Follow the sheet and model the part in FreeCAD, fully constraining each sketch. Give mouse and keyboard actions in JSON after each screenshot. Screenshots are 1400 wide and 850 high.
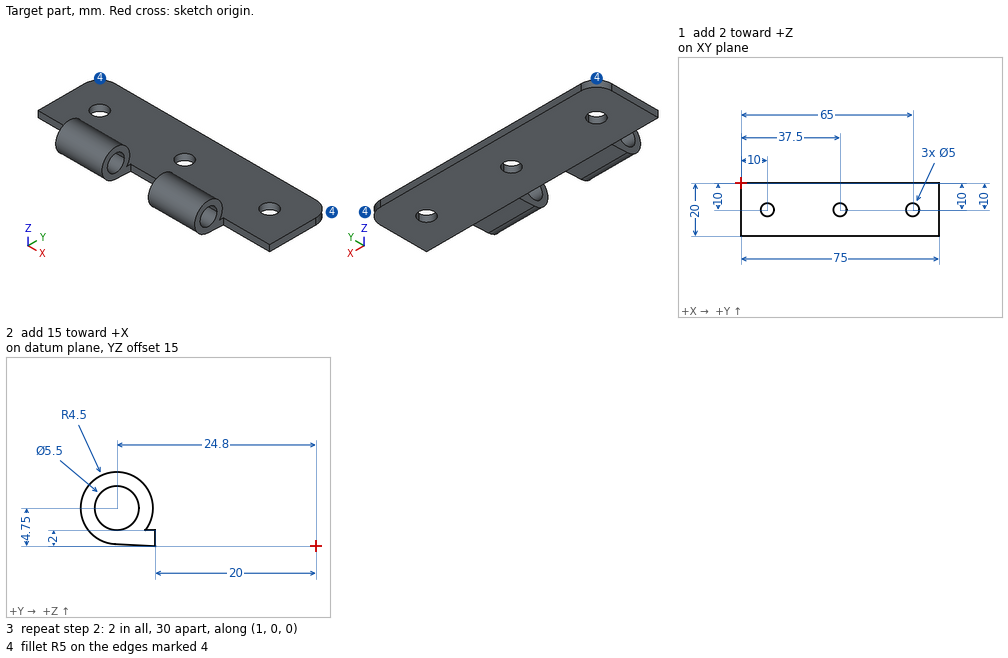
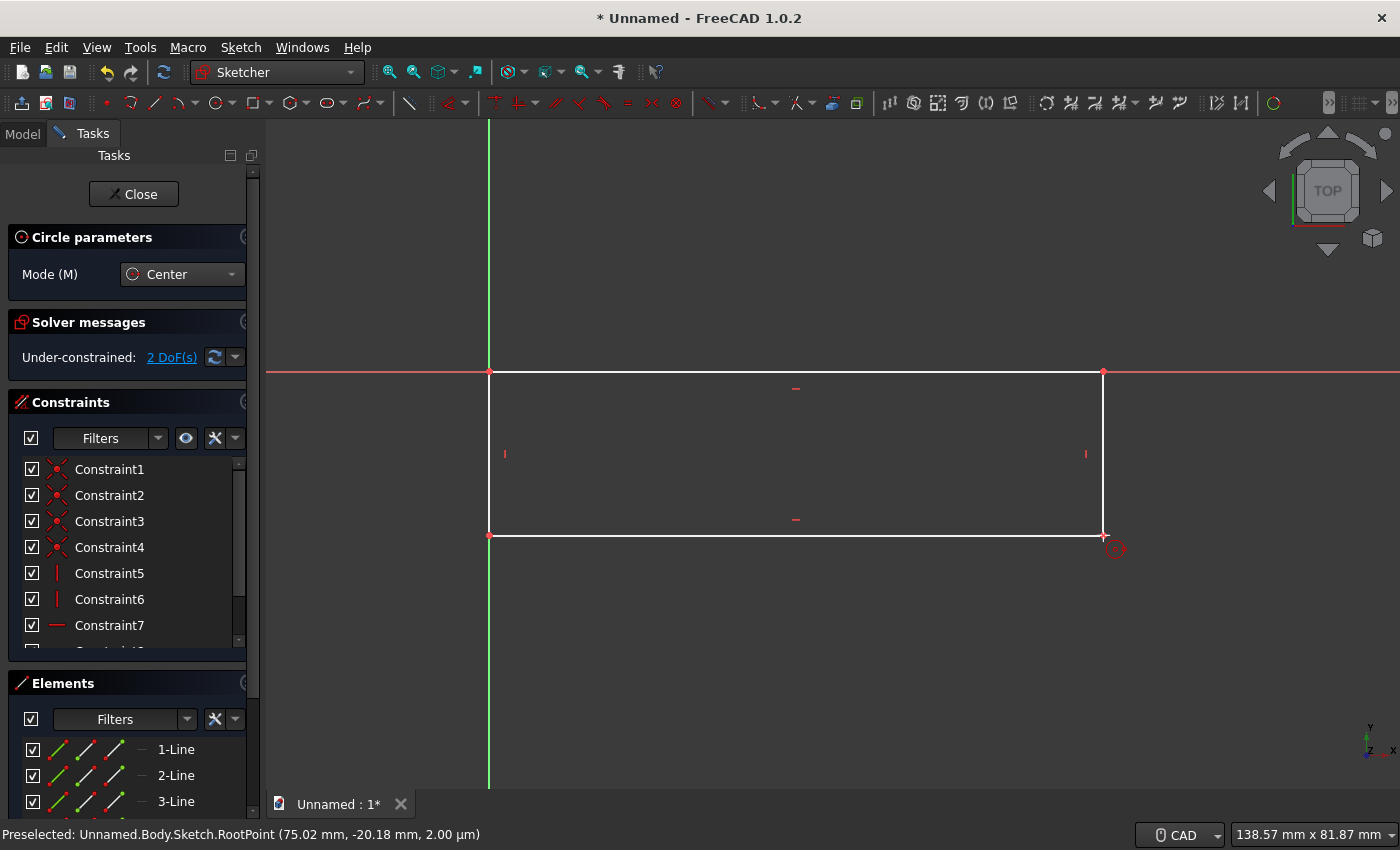
{"action": "left_click", "coordinate": [571, 454]}
{"action": "left_click", "coordinate": [585, 439]}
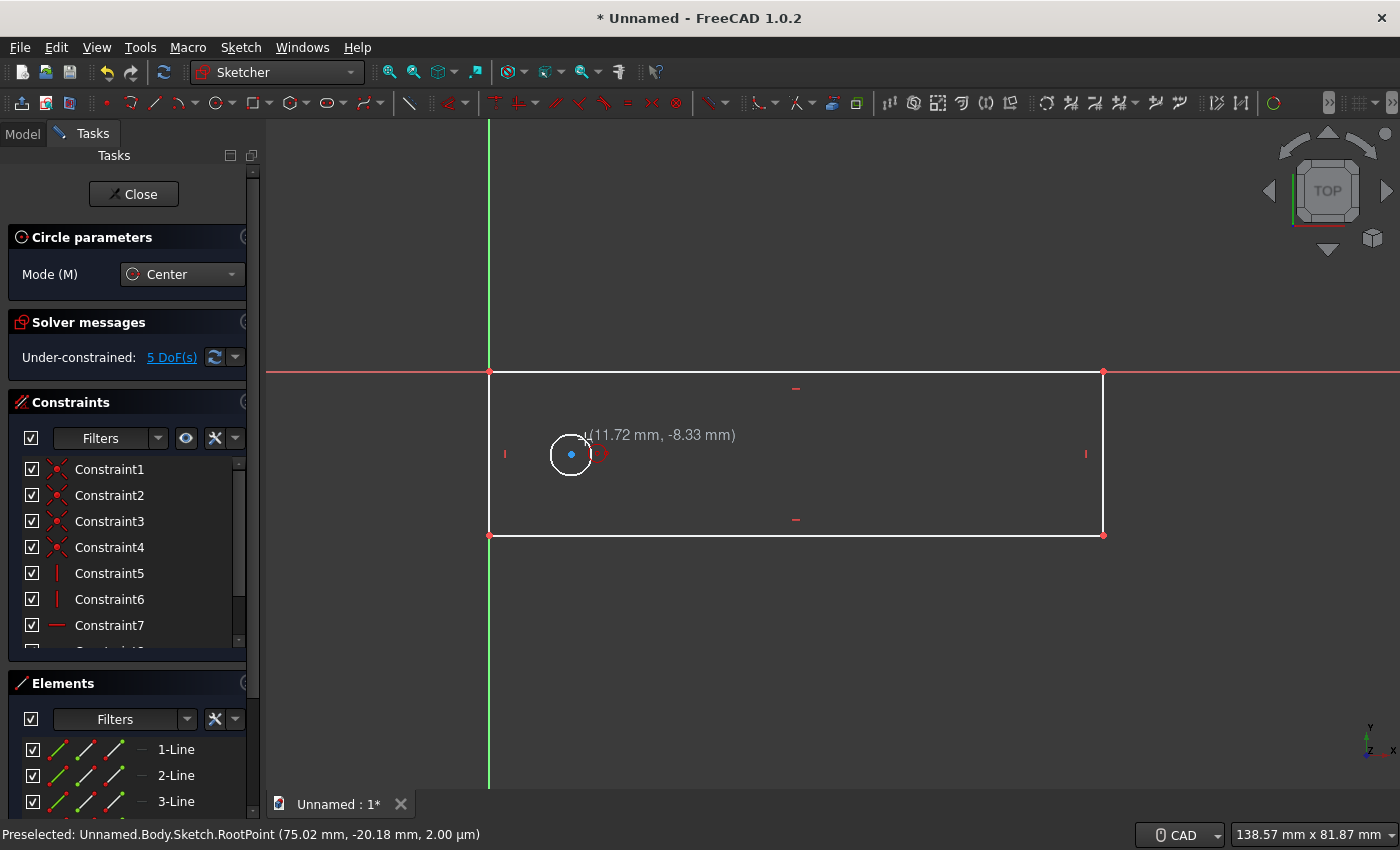
{"action": "left_click", "coordinate": [796, 454]}
{"action": "left_click", "coordinate": [810, 439]}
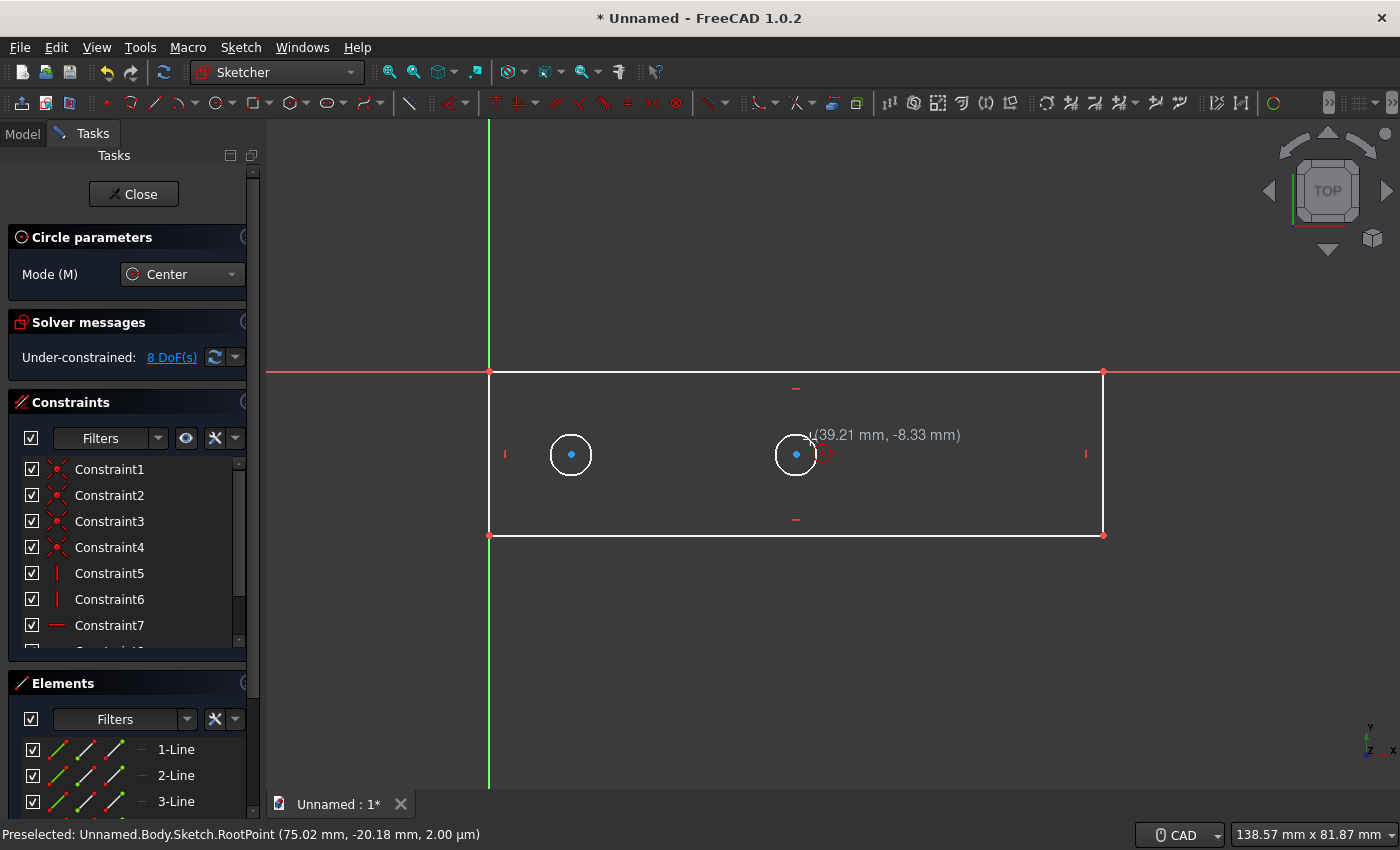
{"action": "left_click", "coordinate": [1021, 454]}
{"action": "left_click", "coordinate": [1036, 439]}
{"action": "key", "text": "Escape"}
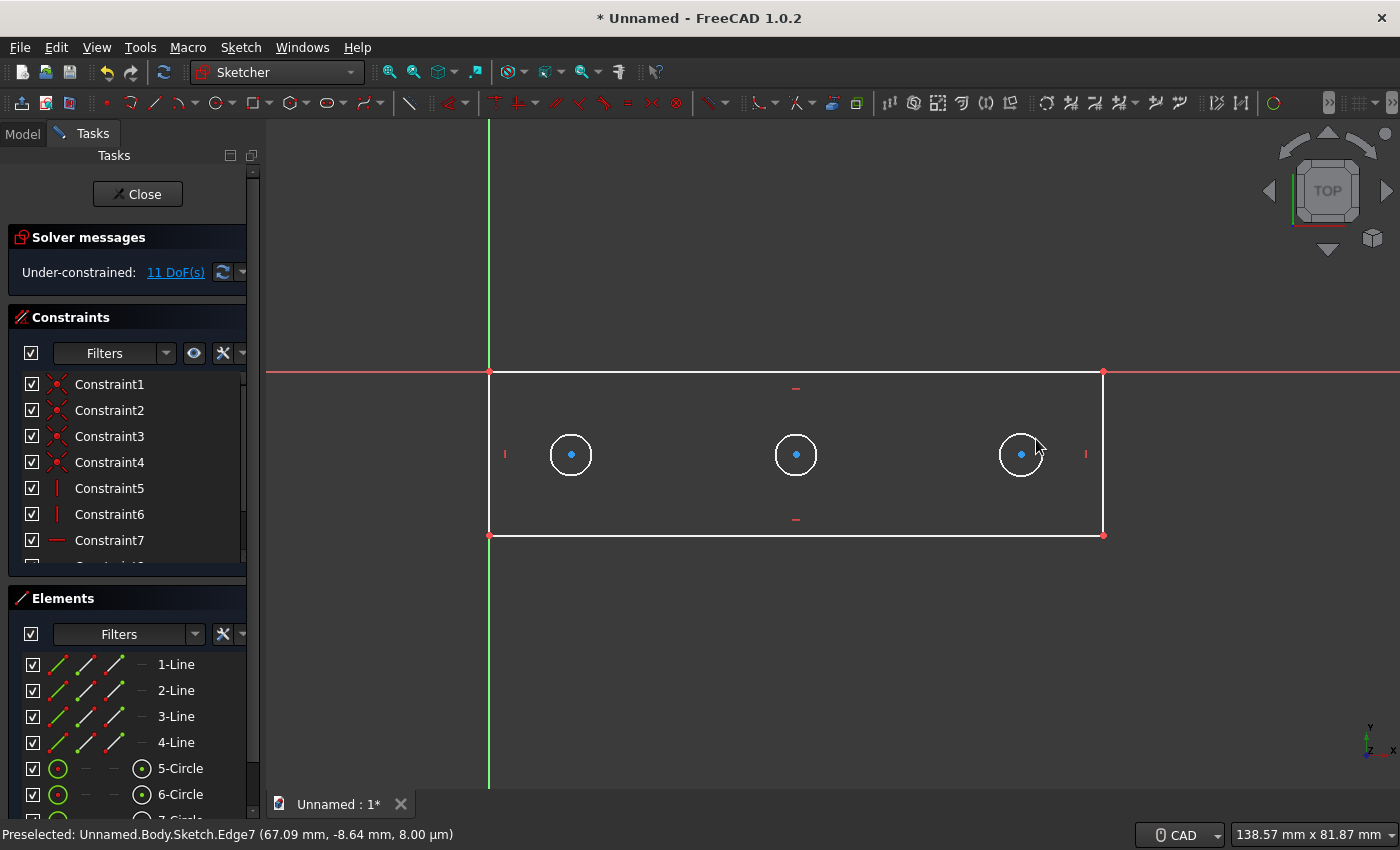
{"action": "left_click", "coordinate": [585, 440]}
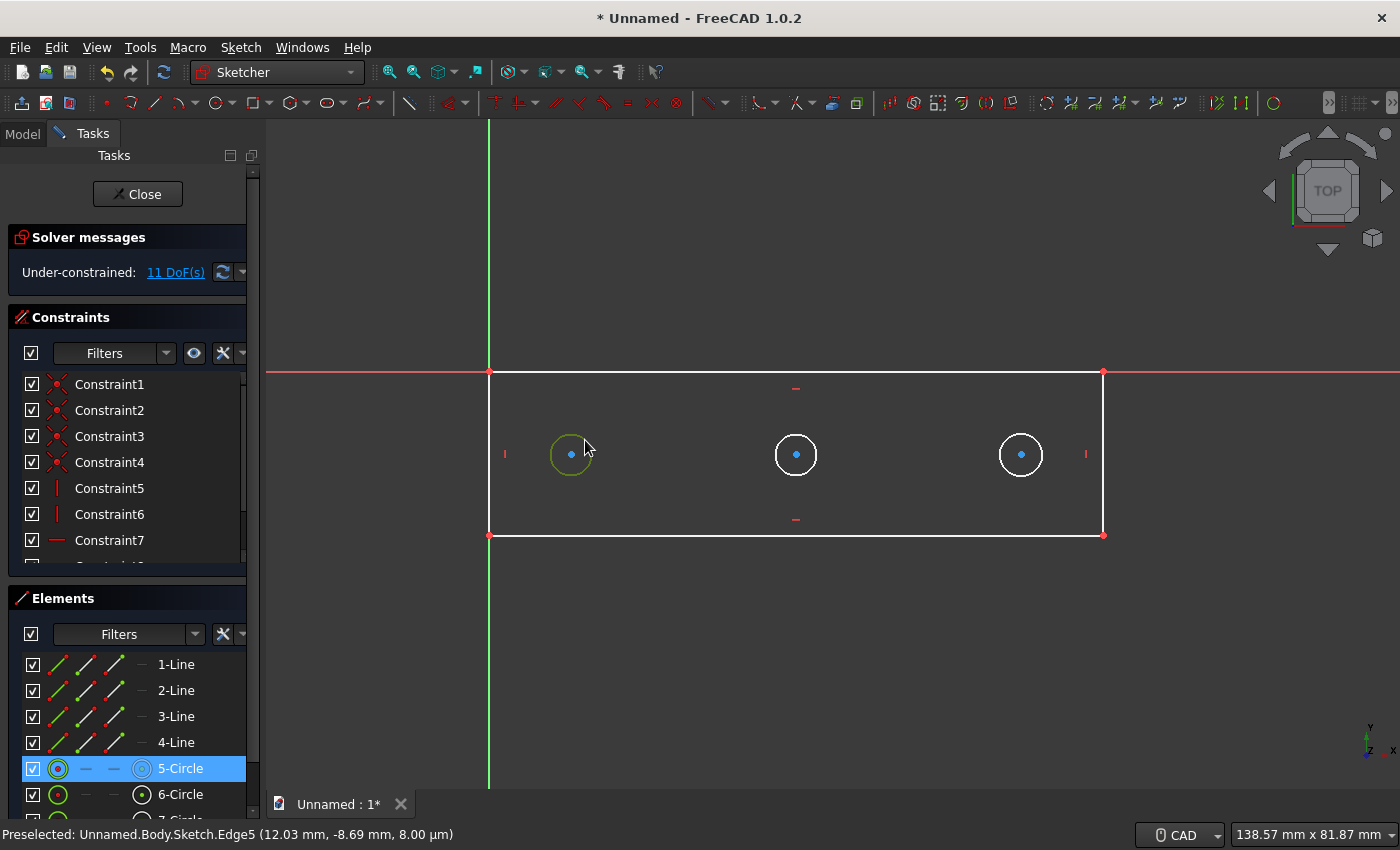
{"action": "left_click", "coordinate": [810, 440]}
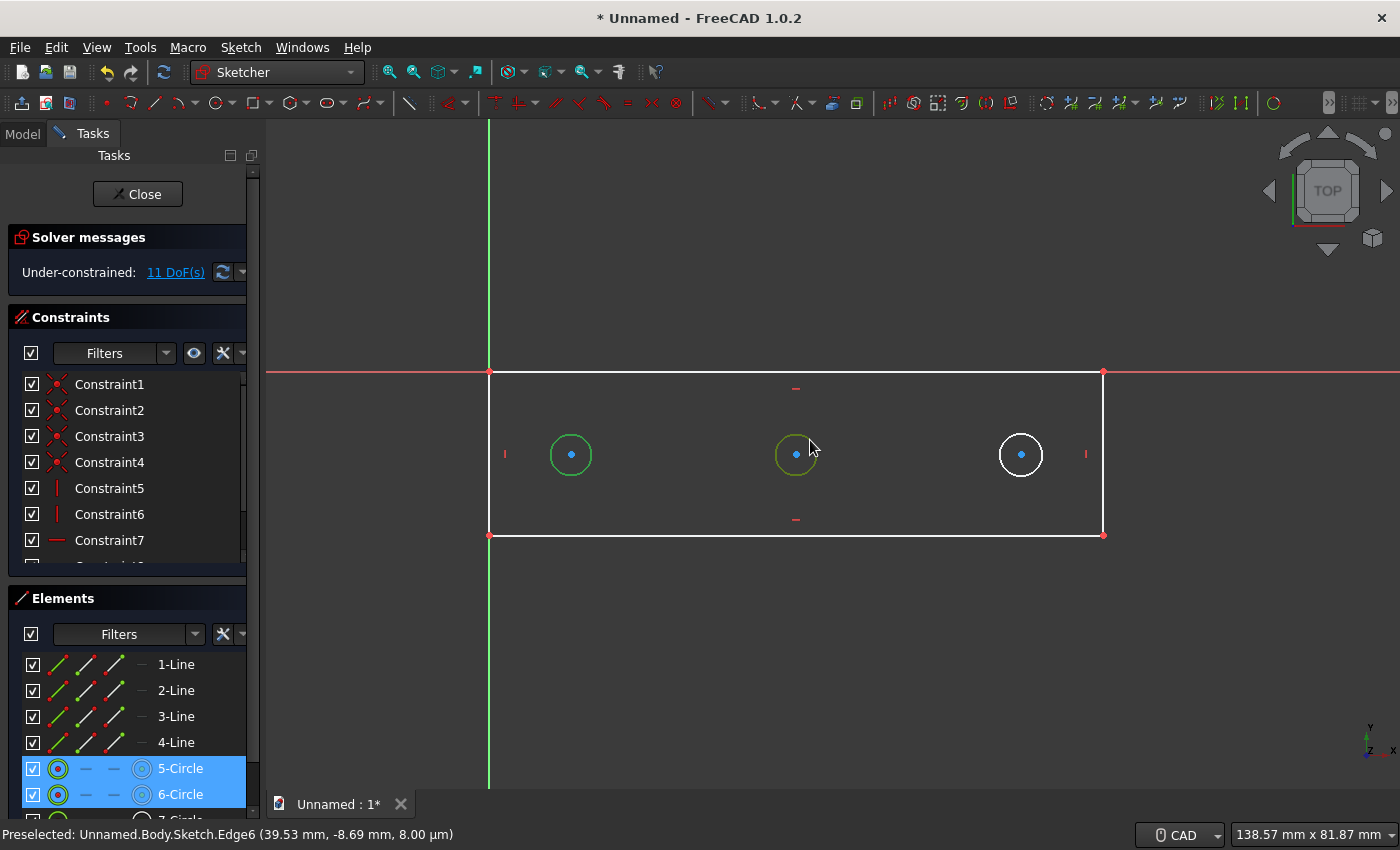
{"action": "left_click", "coordinate": [1036, 440]}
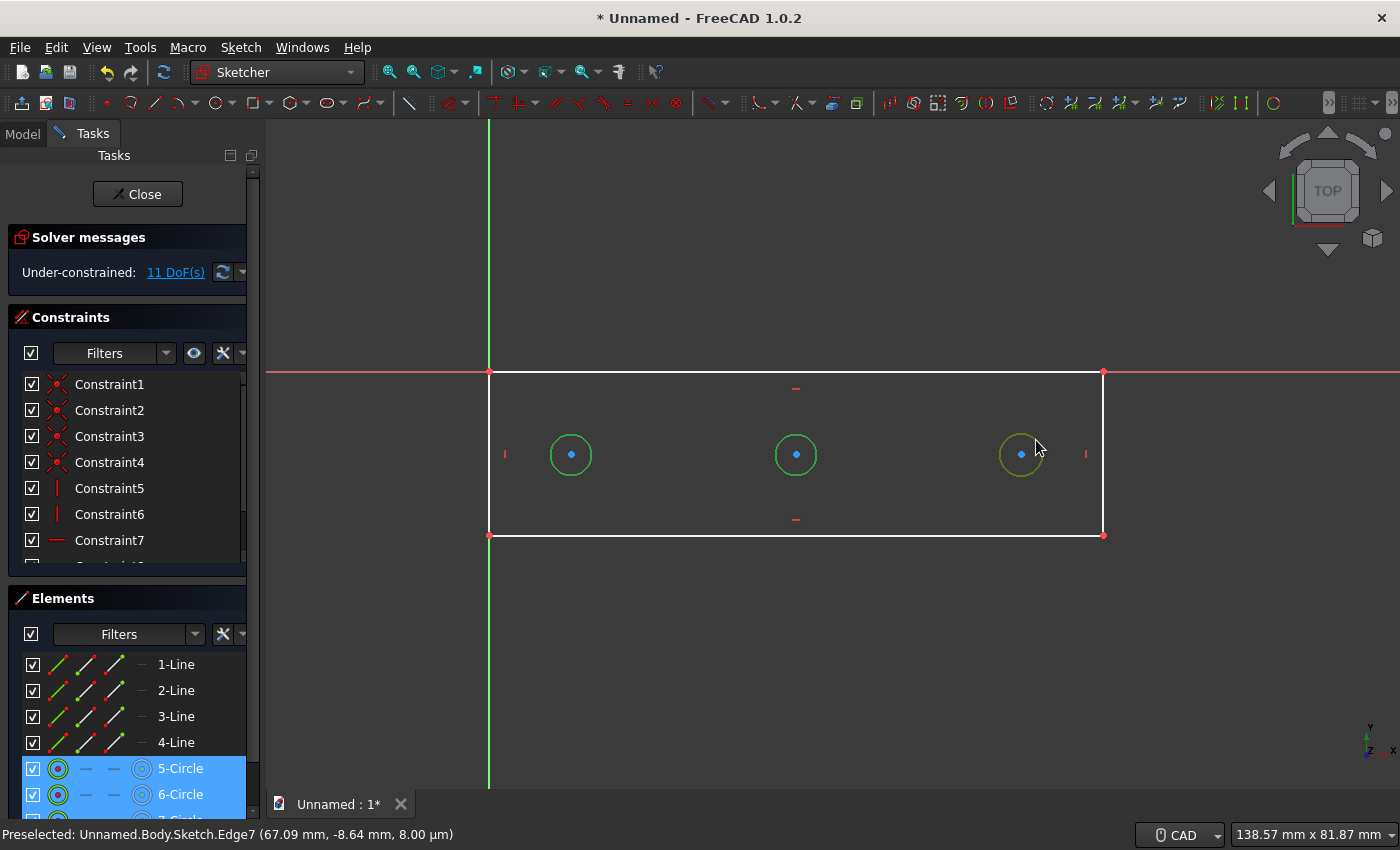
{"action": "key", "text": "e"}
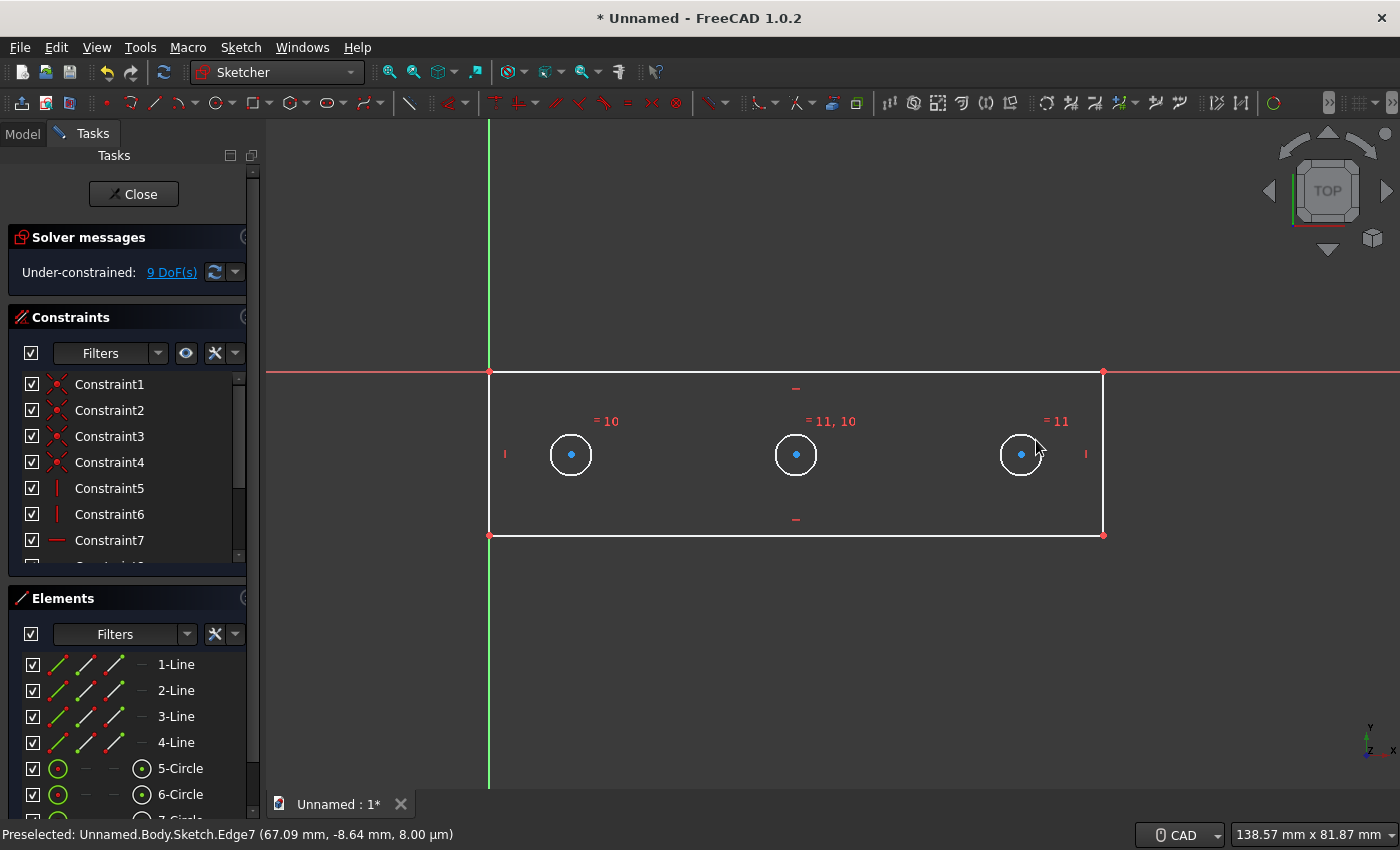
{"action": "left_click", "coordinate": [585, 440]}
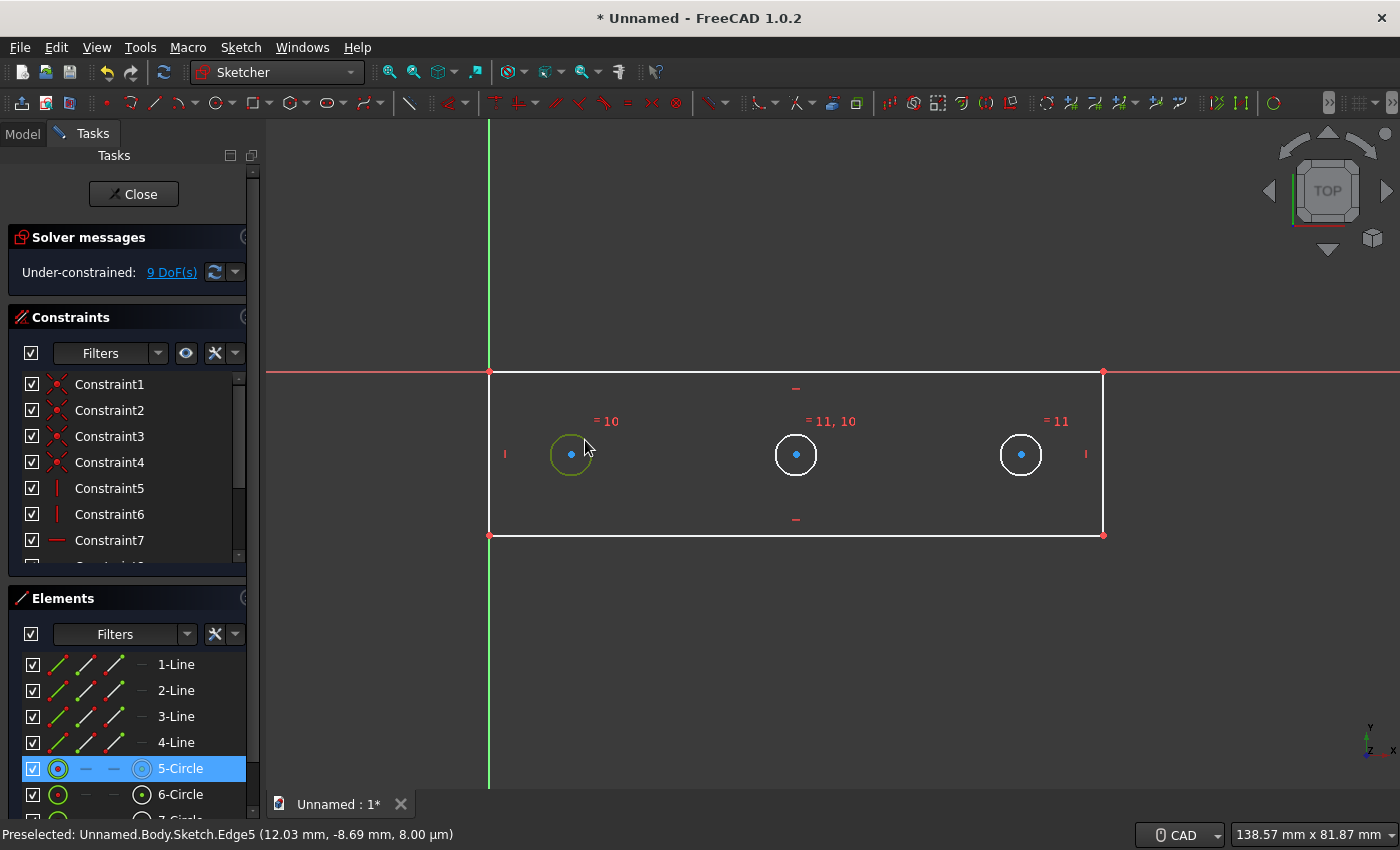
{"action": "left_click", "coordinate": [468, 104]}